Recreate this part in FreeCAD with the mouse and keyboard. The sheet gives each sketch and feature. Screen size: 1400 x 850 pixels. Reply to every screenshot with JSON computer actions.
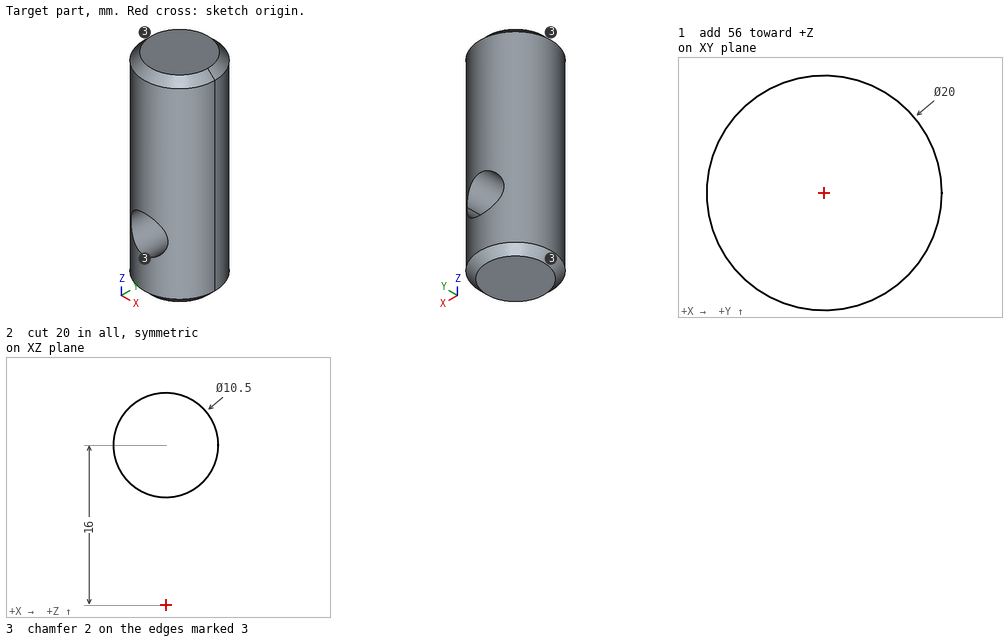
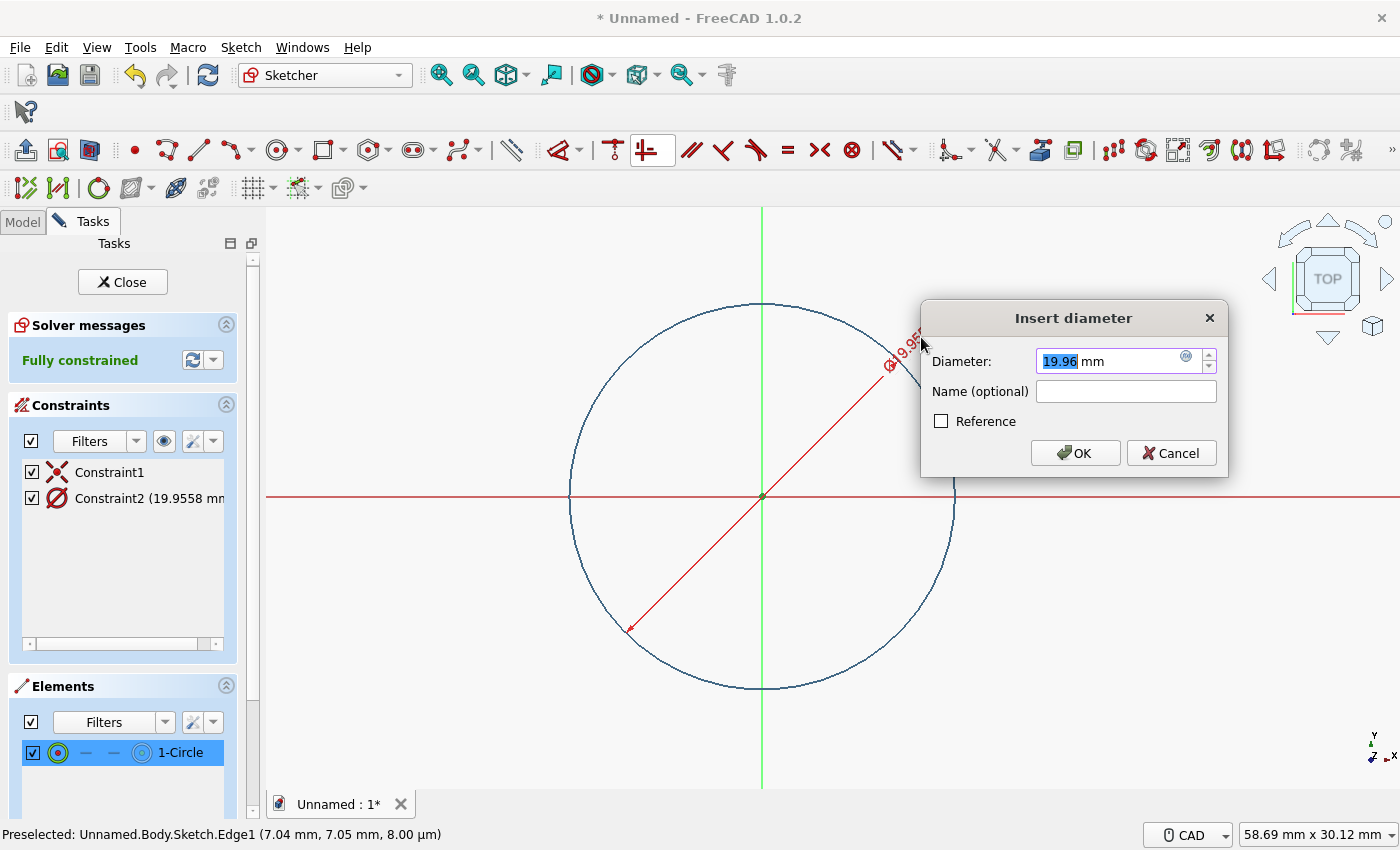
{"action": "type", "text": "20"}
{"action": "key", "text": "Return"}
{"action": "key", "text": "Escape"}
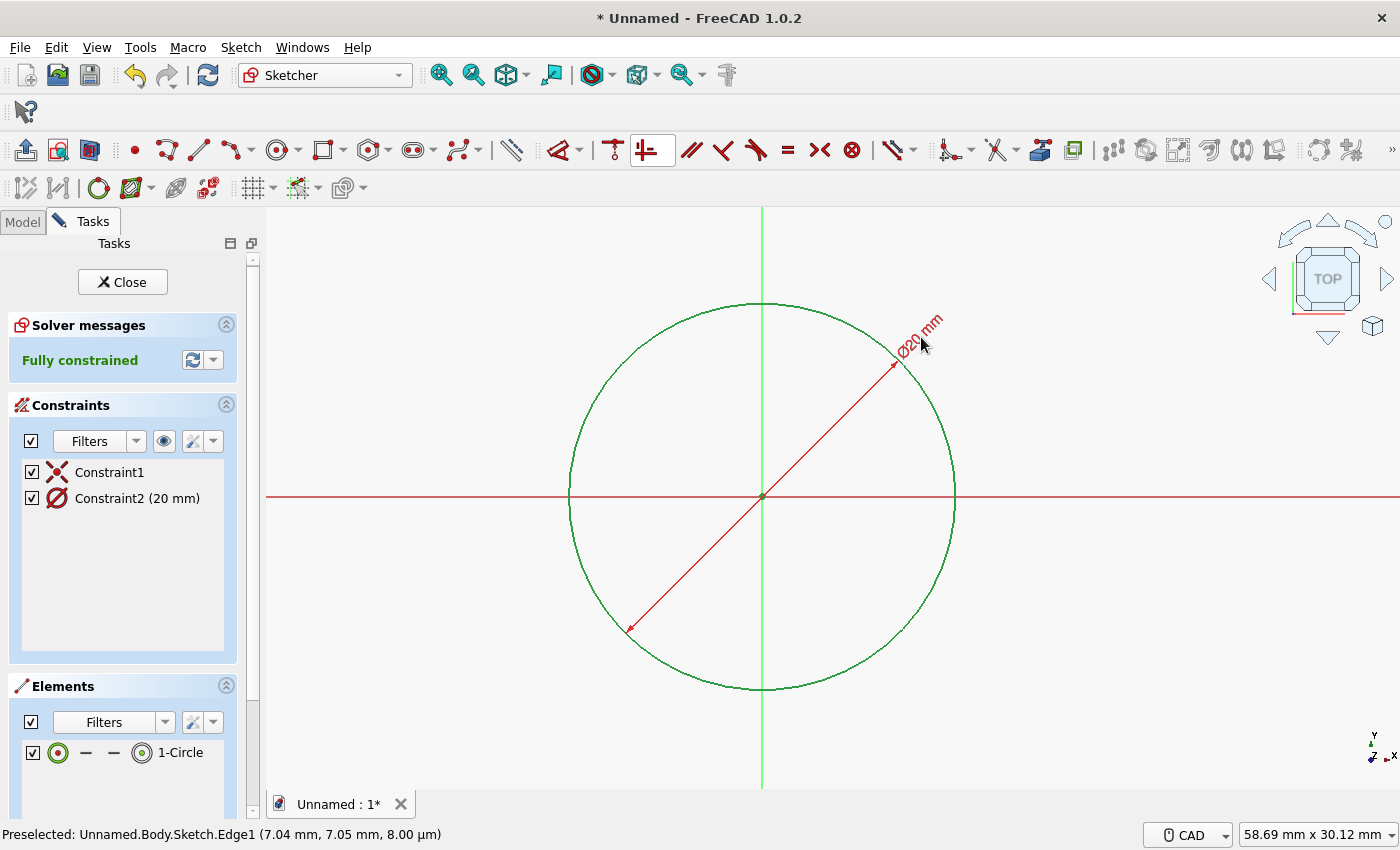
{"action": "left_click", "coordinate": [123, 282]}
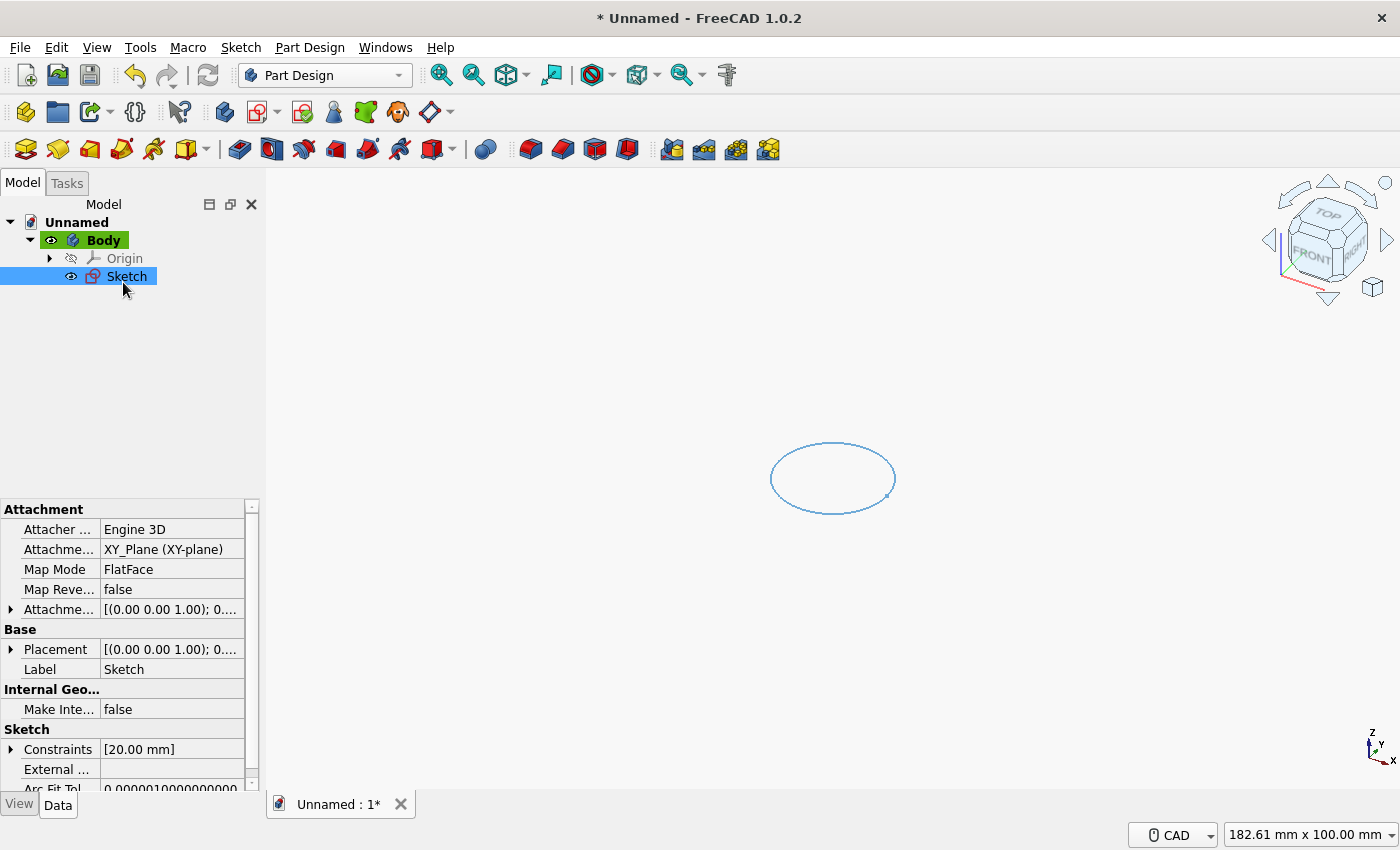
{"action": "left_click", "coordinate": [26, 150]}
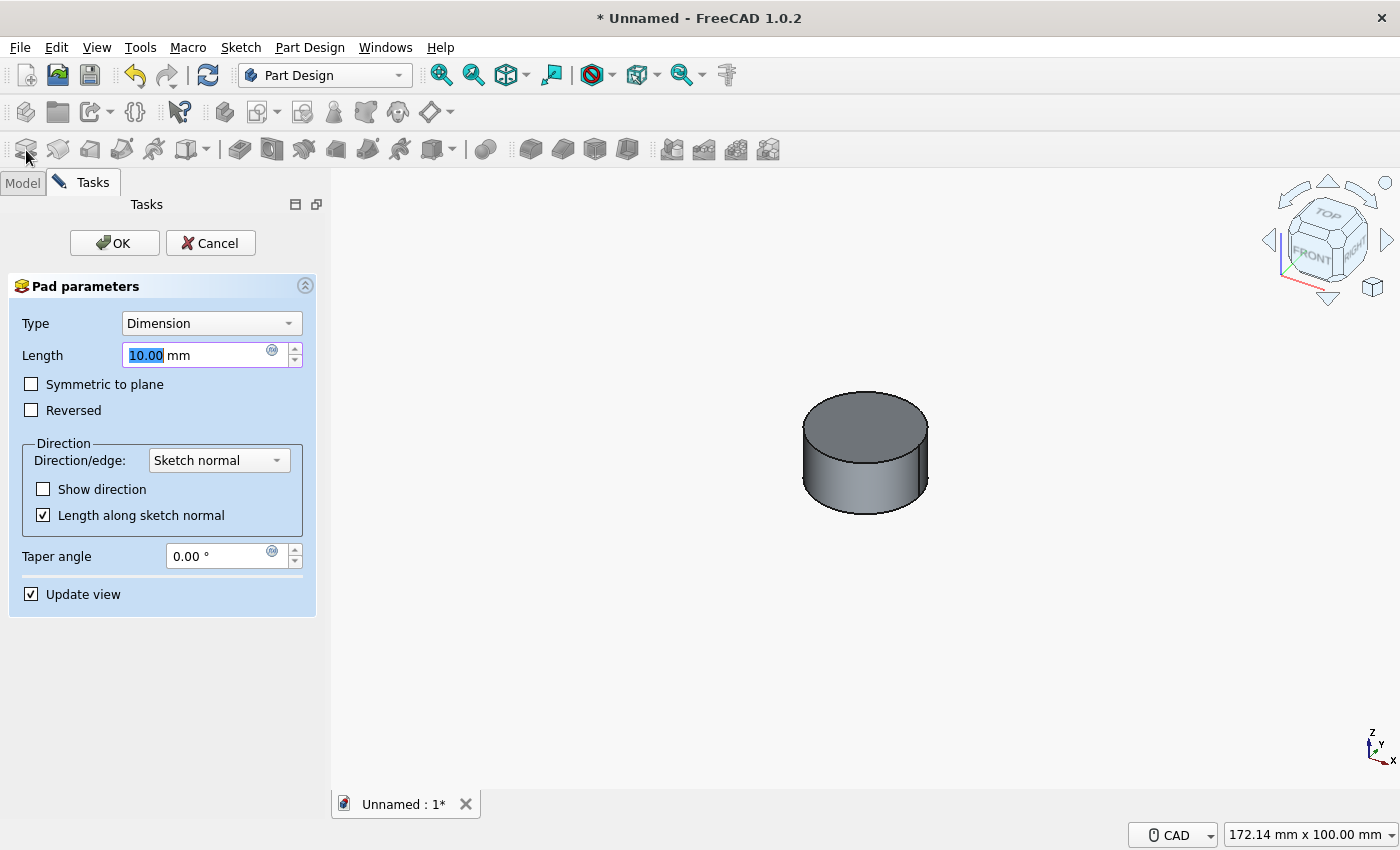
{"action": "type", "text": "56"}
{"action": "key", "text": "Tab"}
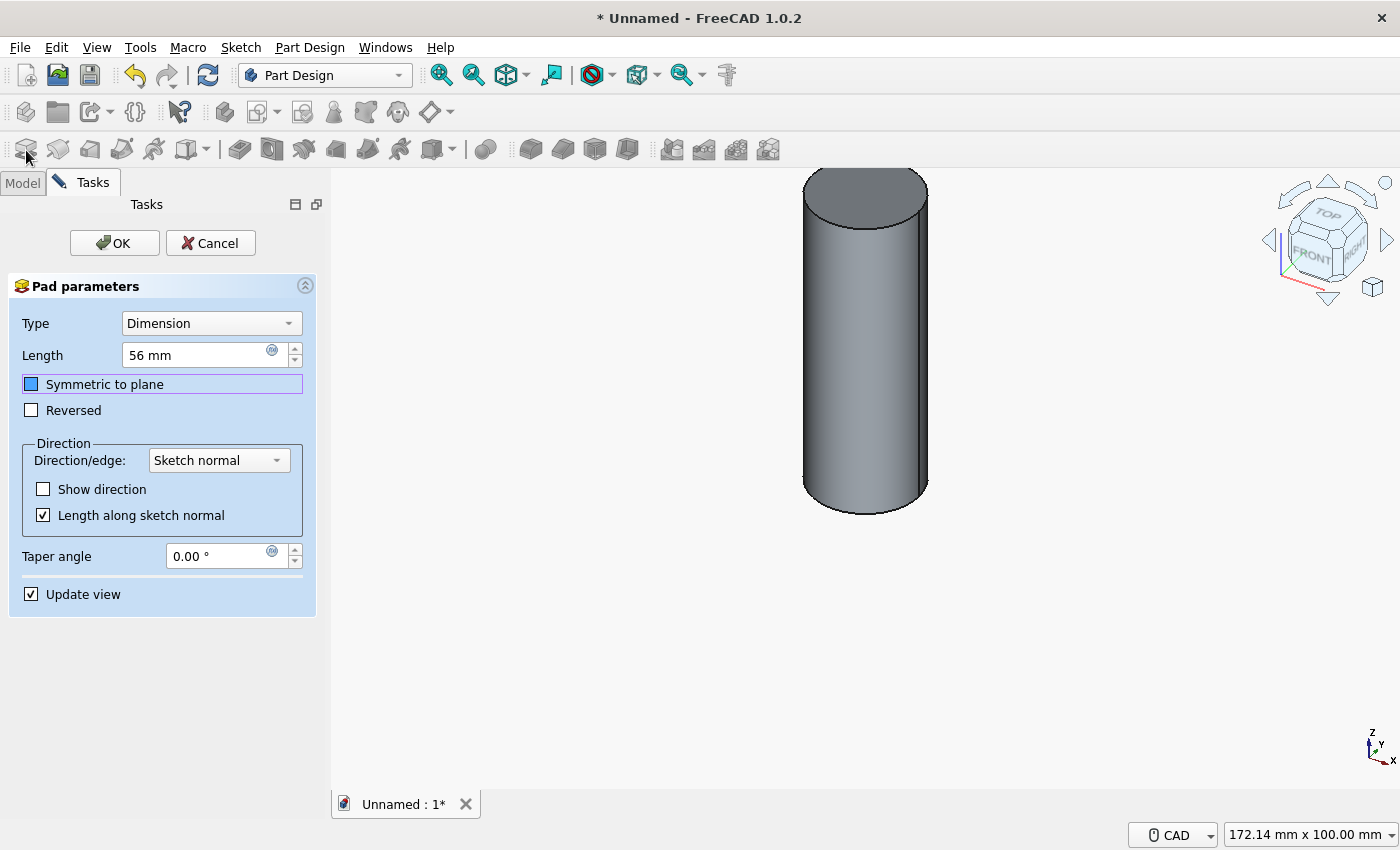
{"action": "left_click", "coordinate": [115, 243]}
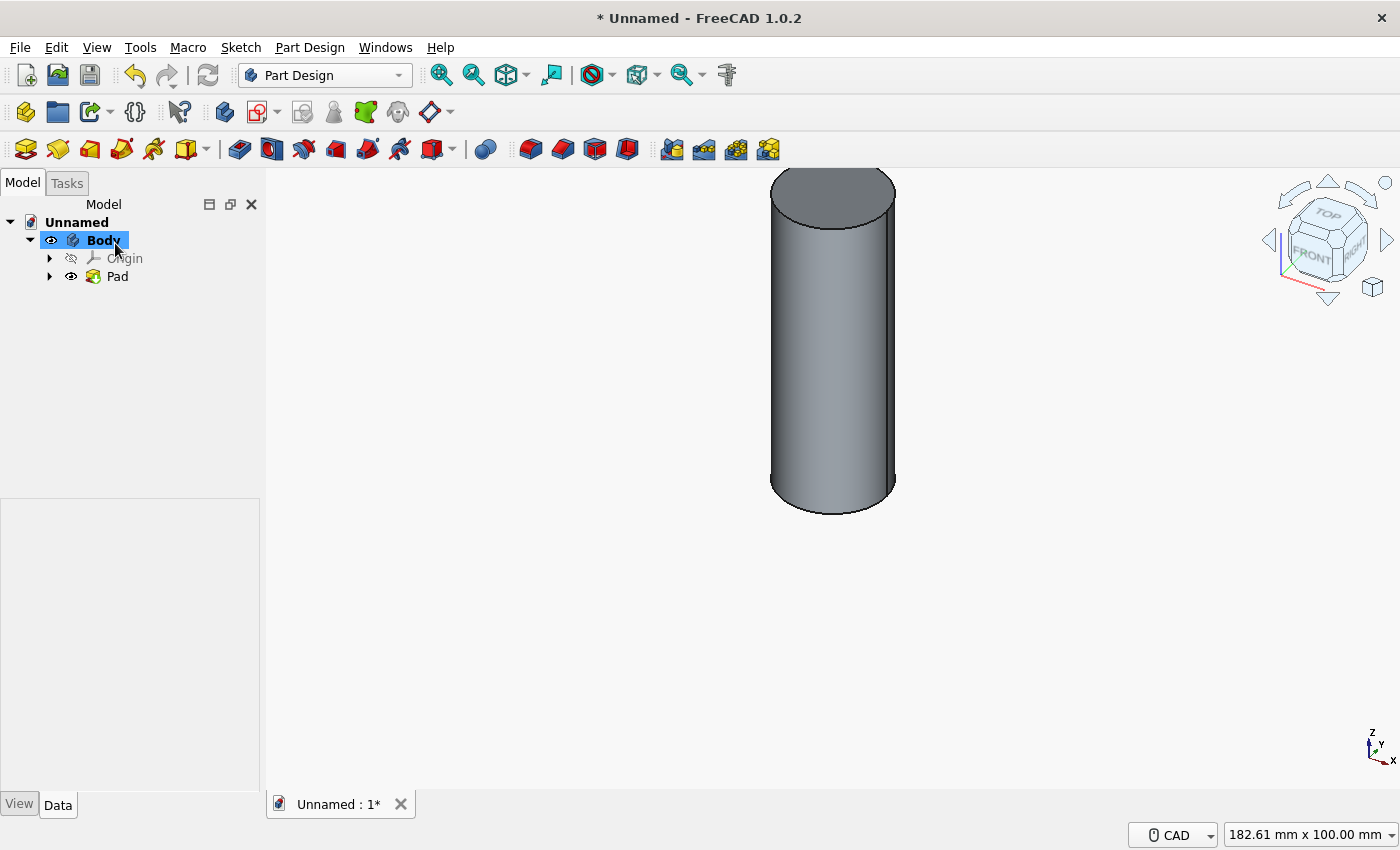
{"action": "left_click", "coordinate": [442, 76]}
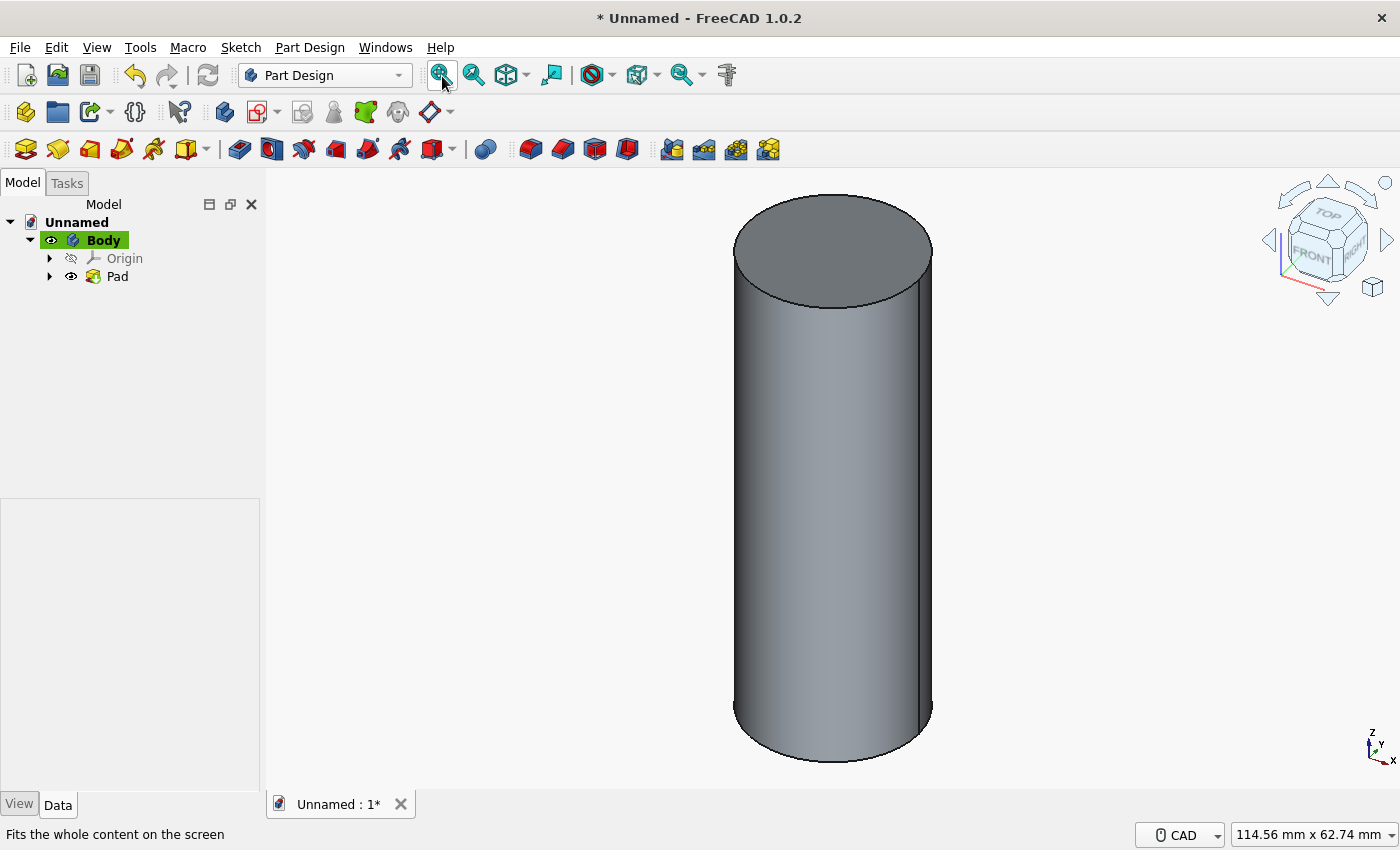
{"action": "left_click", "coordinate": [258, 112]}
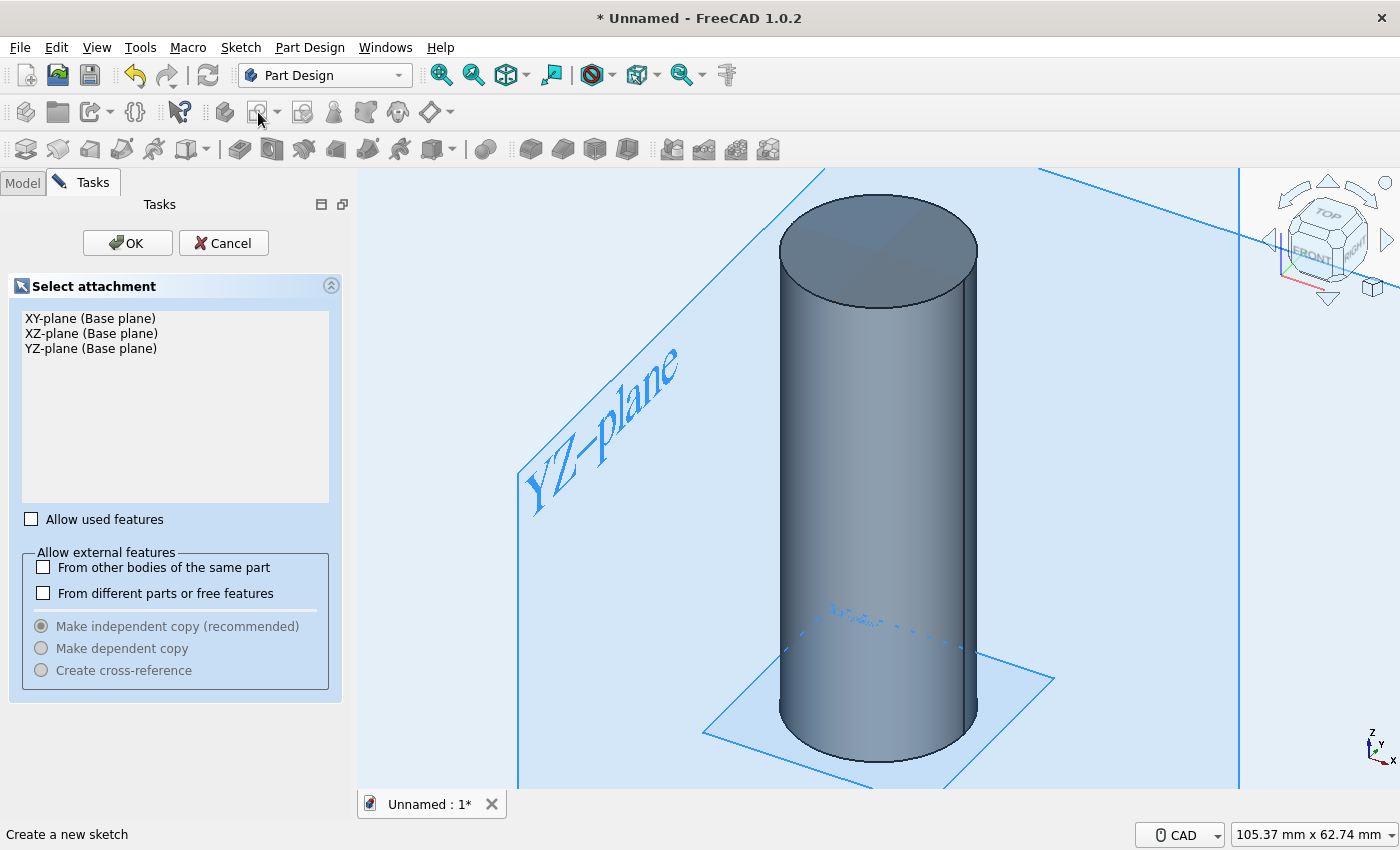
{"action": "left_click", "coordinate": [82, 334]}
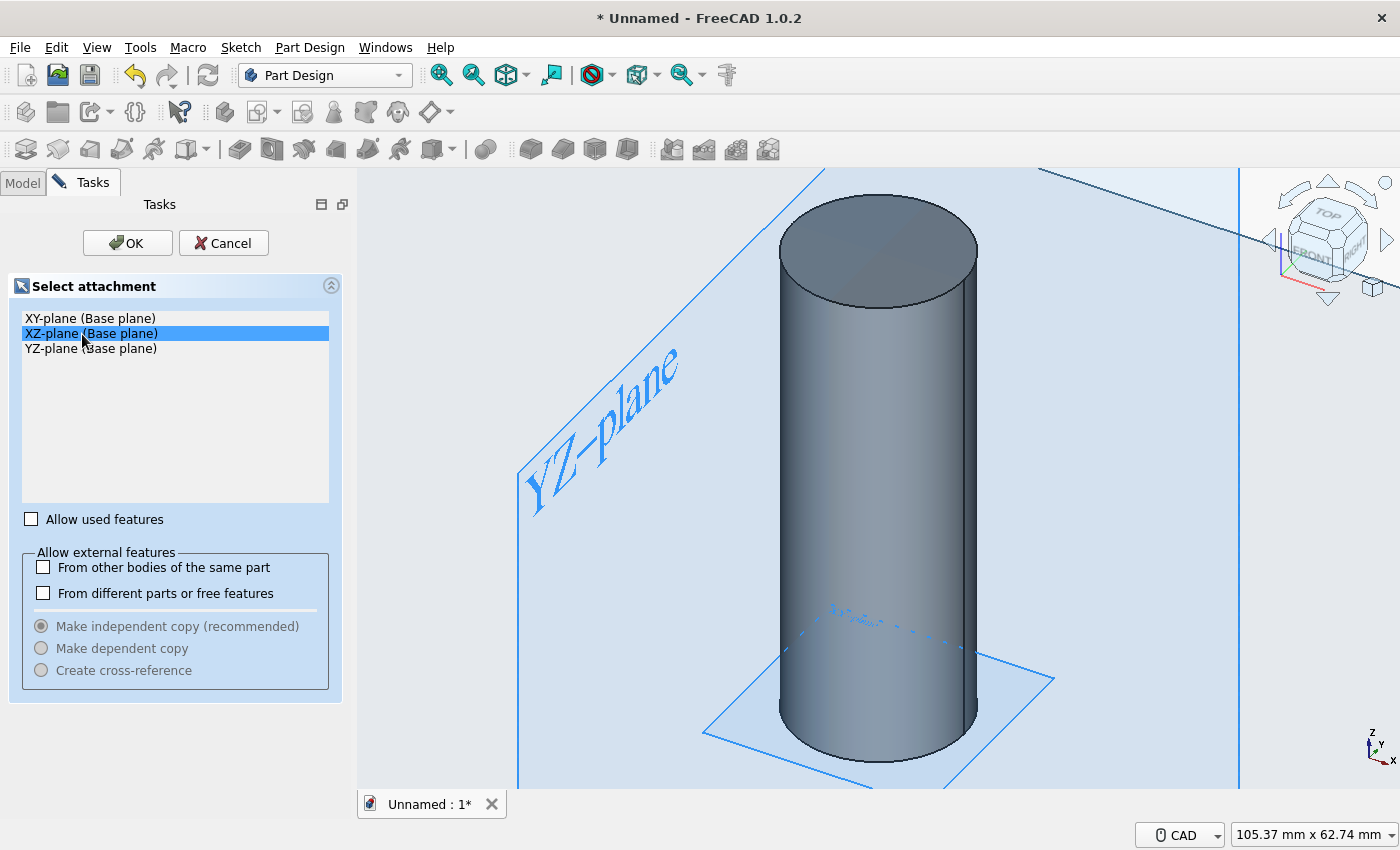
{"action": "left_click", "coordinate": [128, 243]}